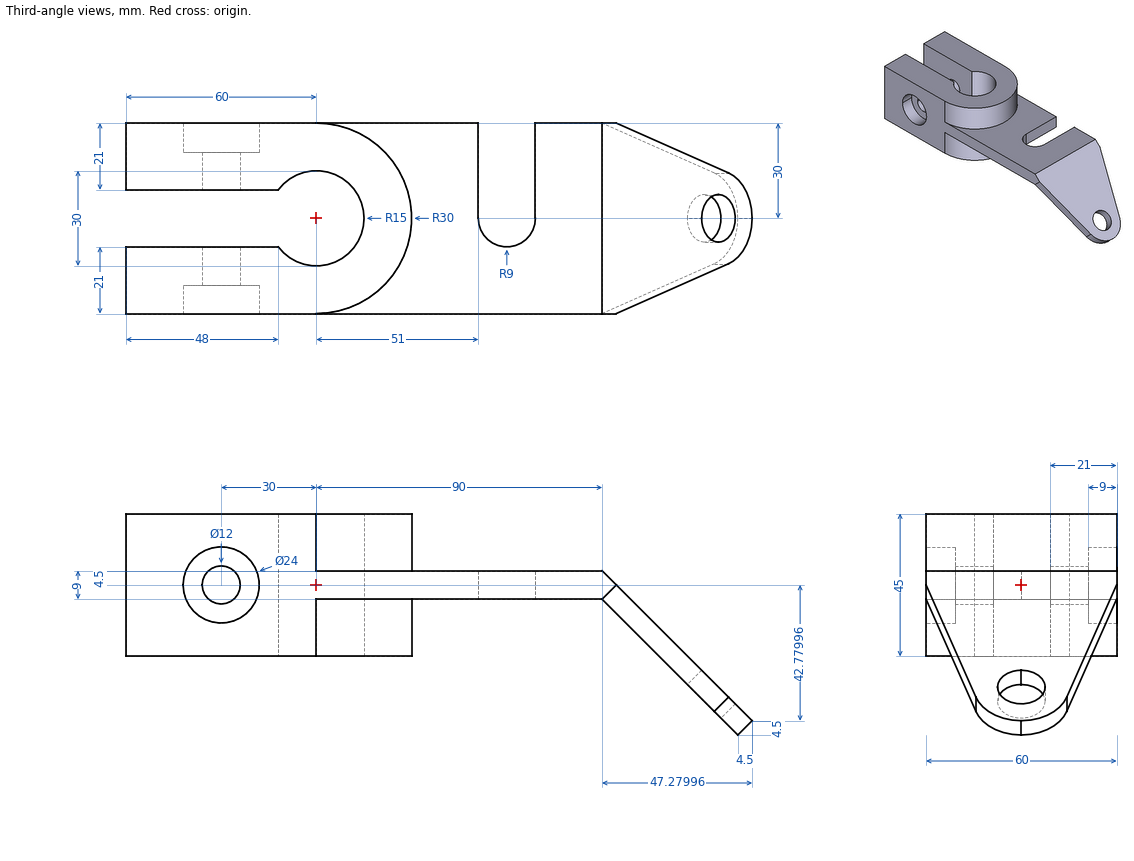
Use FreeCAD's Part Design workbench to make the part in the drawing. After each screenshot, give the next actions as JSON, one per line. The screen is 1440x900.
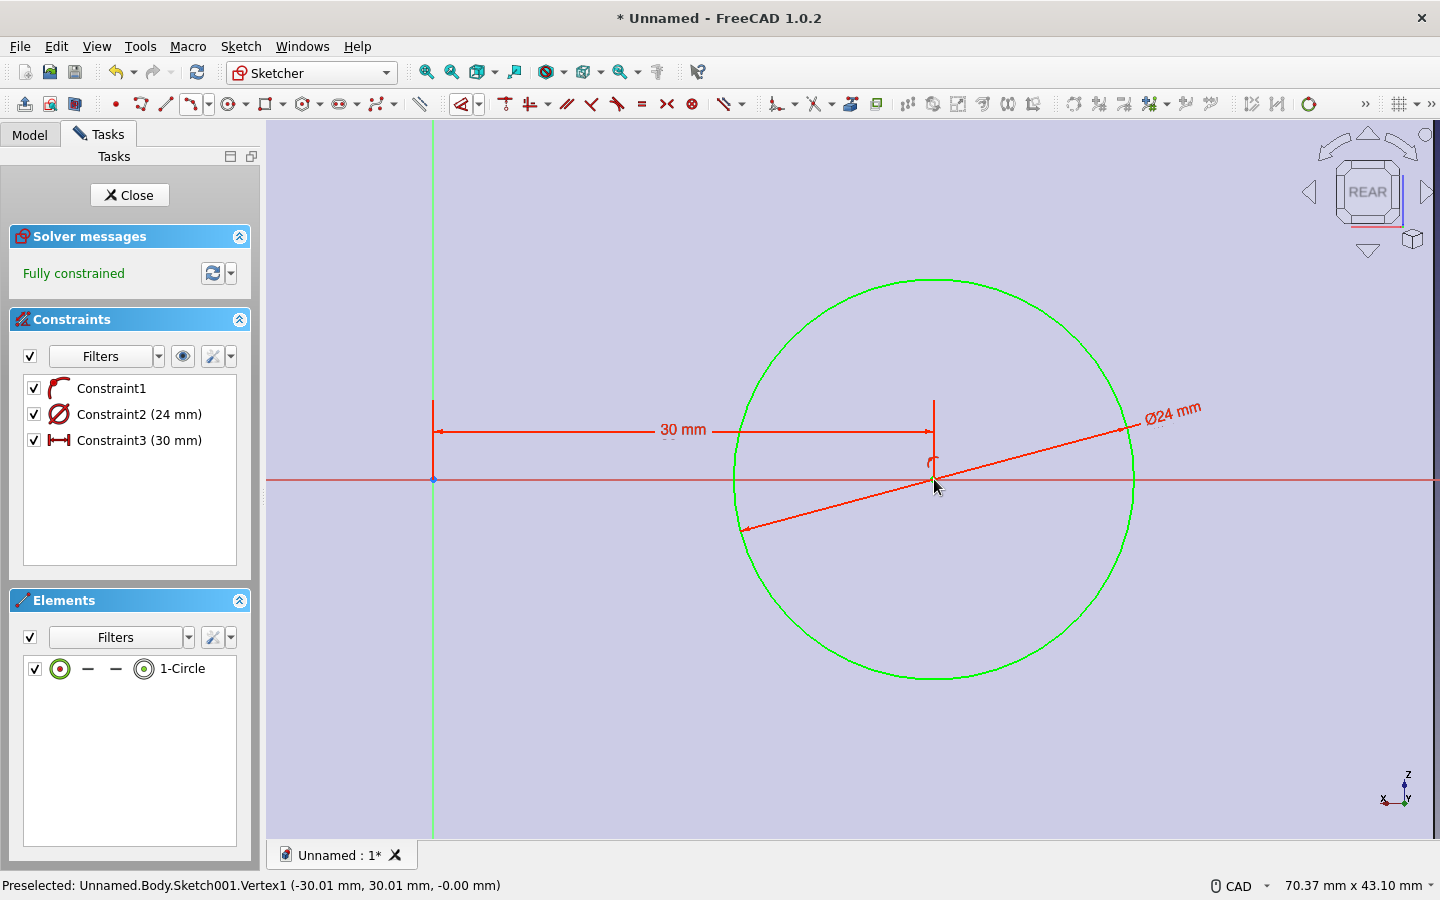
{"action": "left_click", "coordinate": [130, 195]}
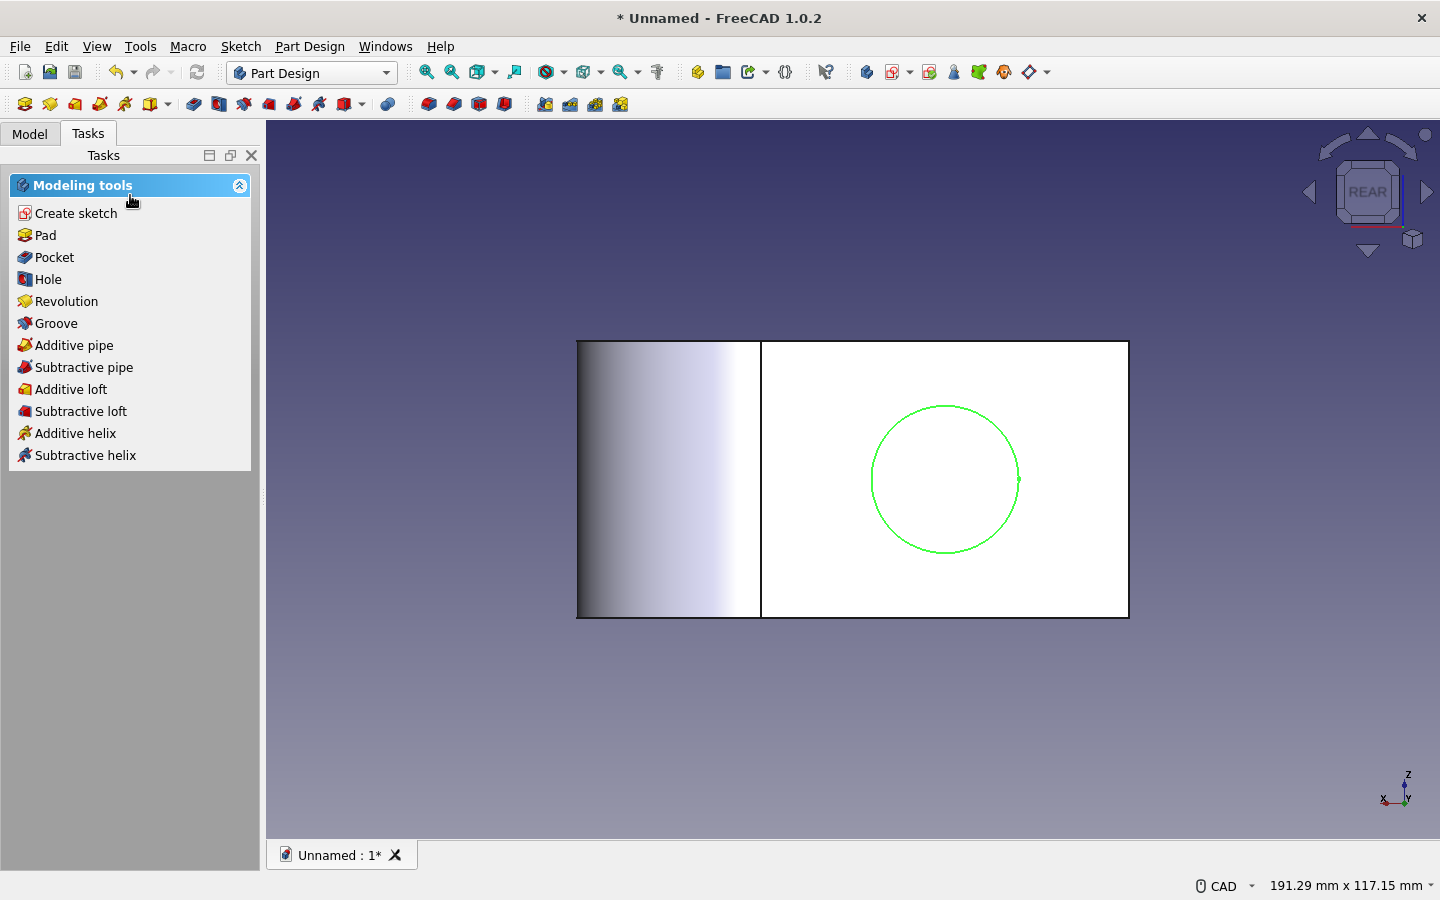
{"action": "left_click", "coordinate": [194, 104]}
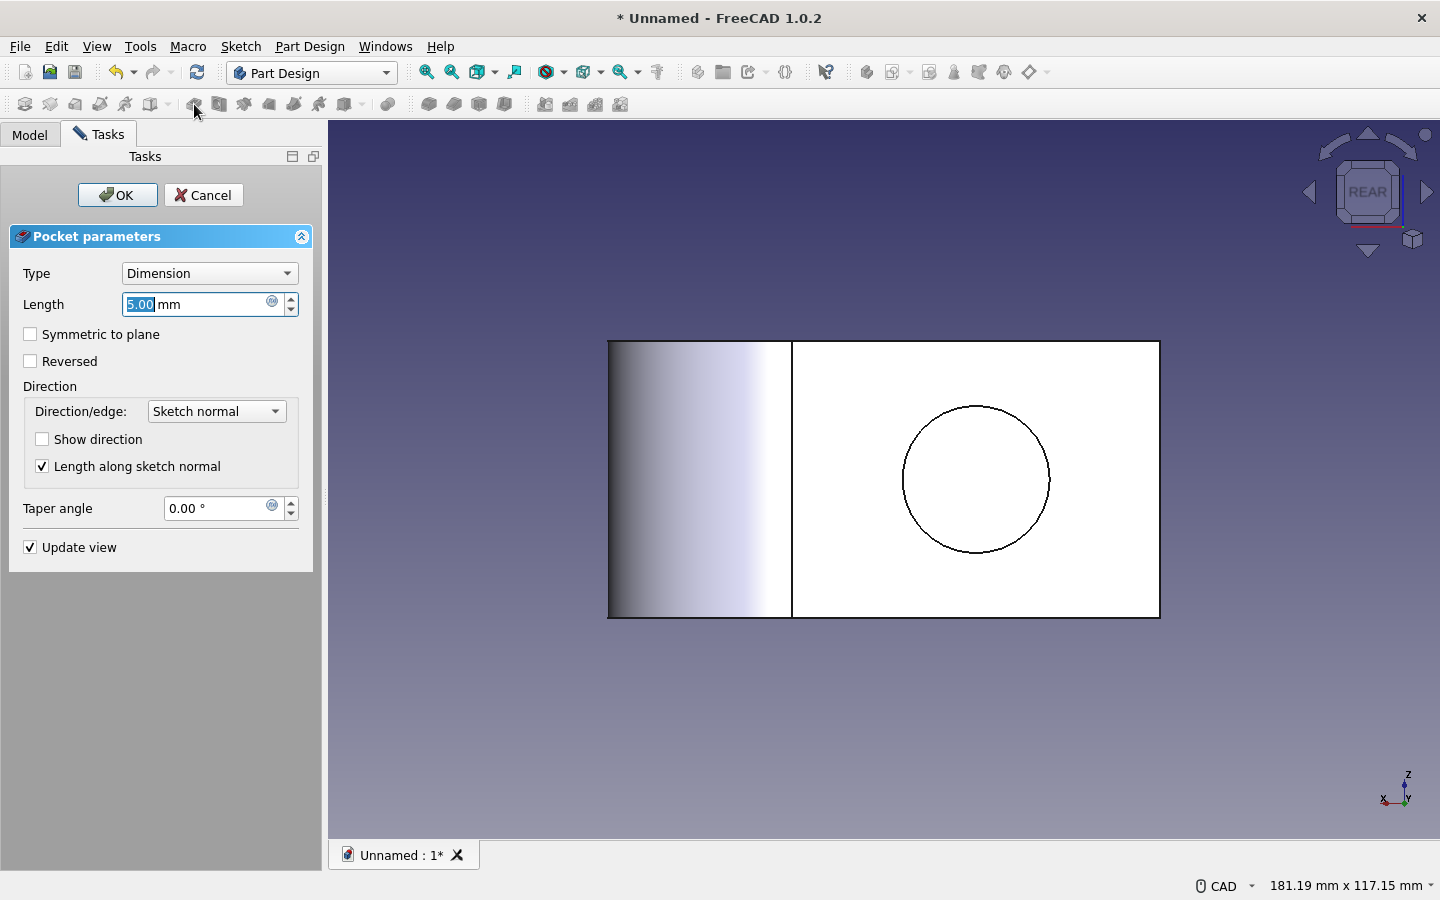
{"action": "type", "text": "9"}
{"action": "key", "text": "Tab"}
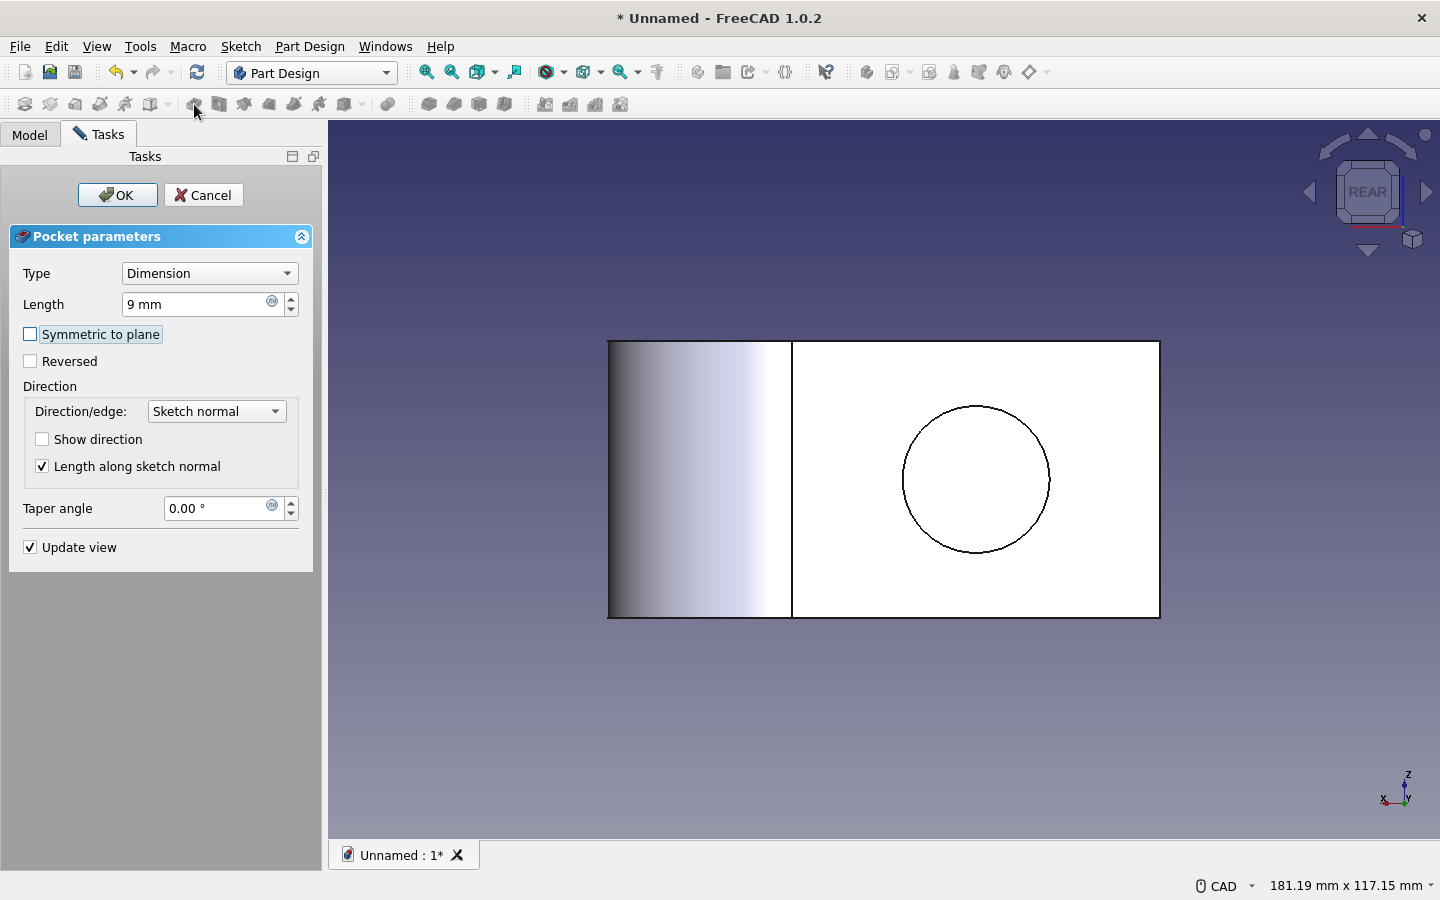
{"action": "left_click", "coordinate": [118, 195]}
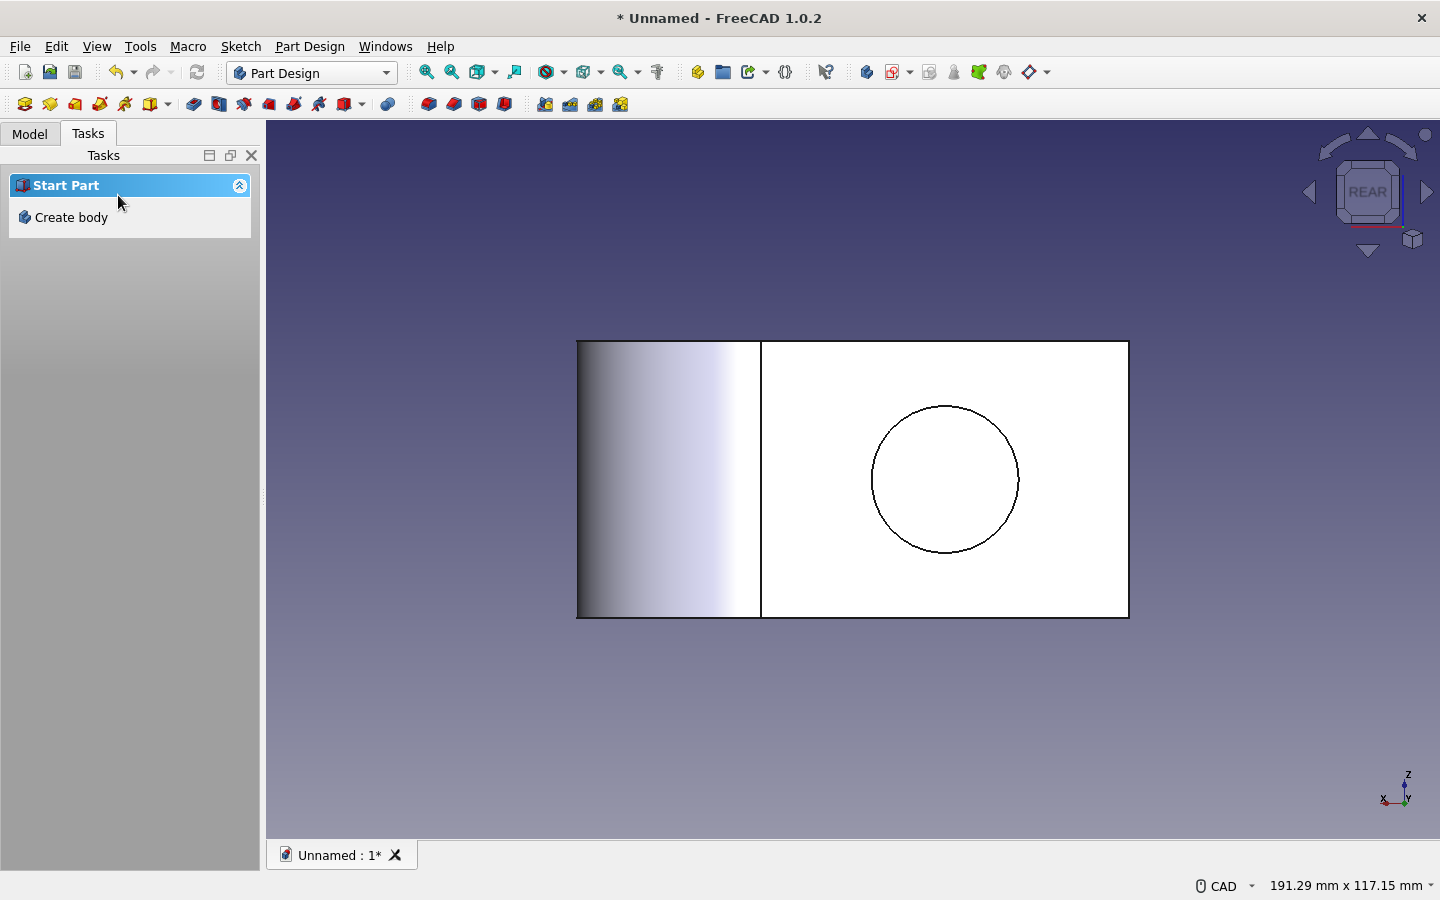
{"action": "left_click", "coordinate": [840, 400]}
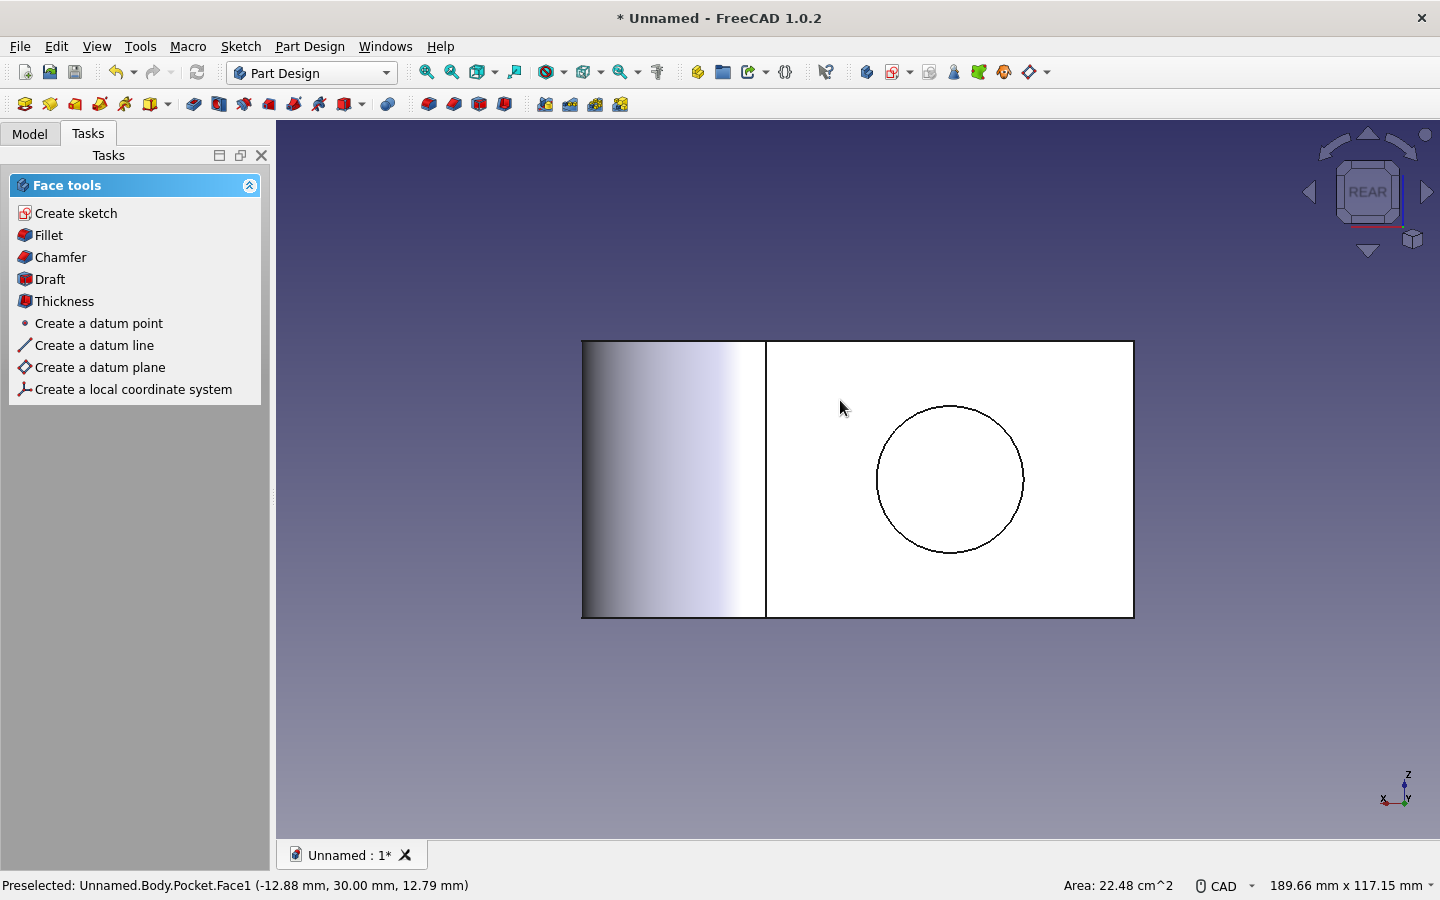
{"action": "left_click", "coordinate": [892, 72]}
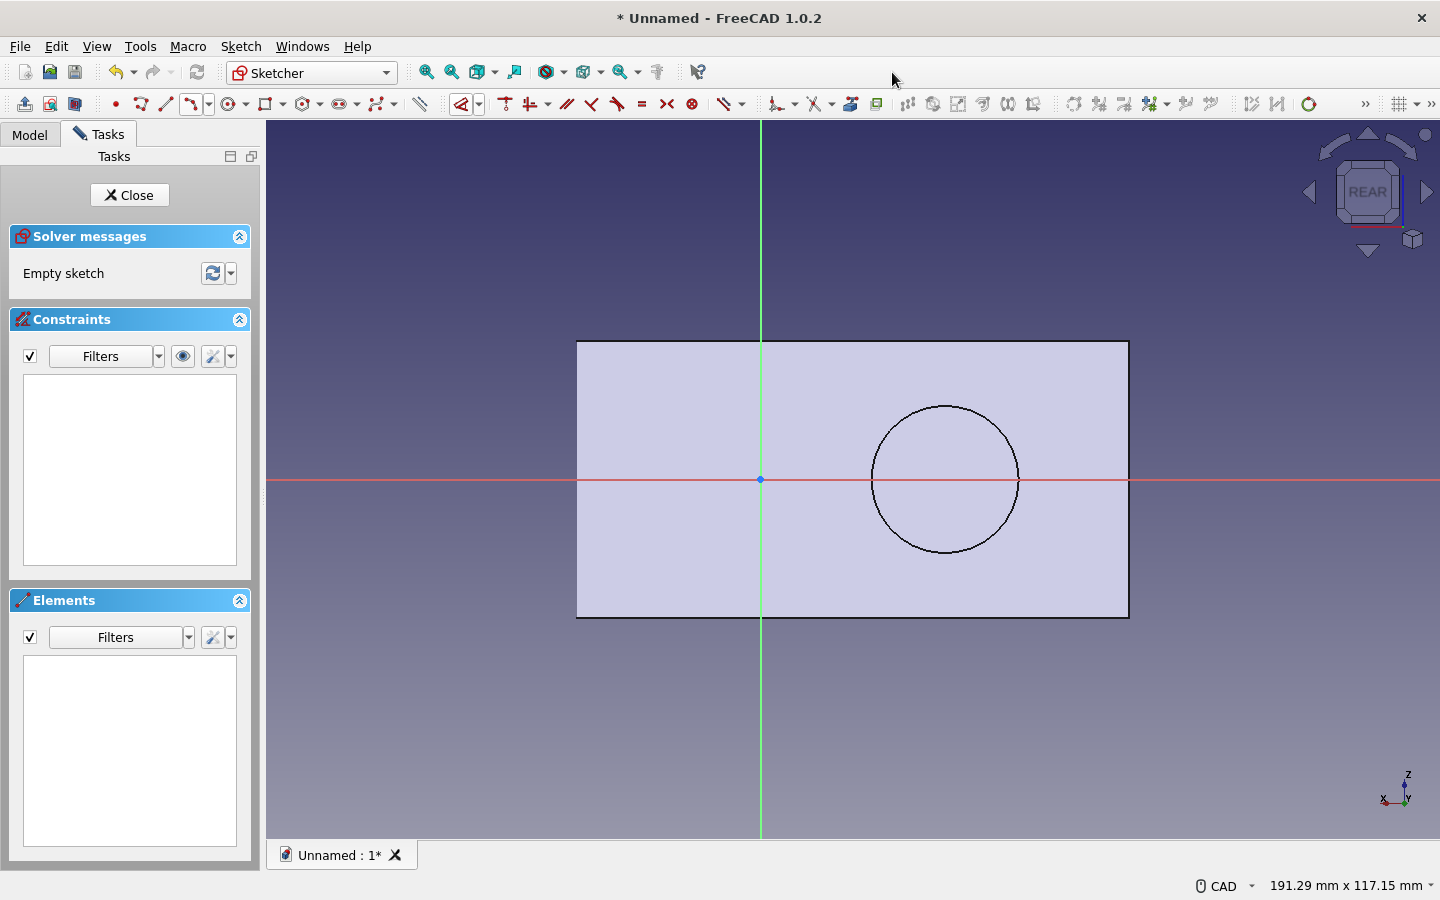
{"action": "scroll", "coordinate": [977, 480], "scroll_direction": "up", "scroll_amount": 9}